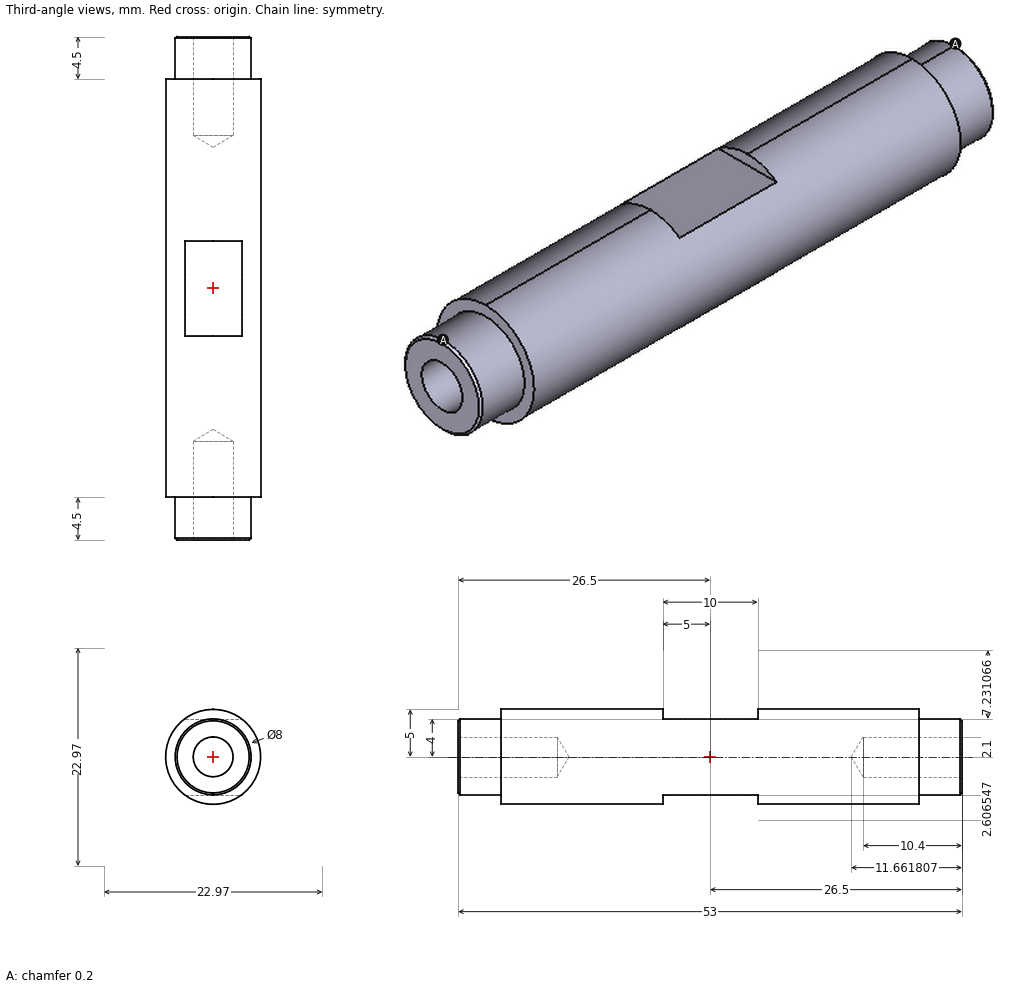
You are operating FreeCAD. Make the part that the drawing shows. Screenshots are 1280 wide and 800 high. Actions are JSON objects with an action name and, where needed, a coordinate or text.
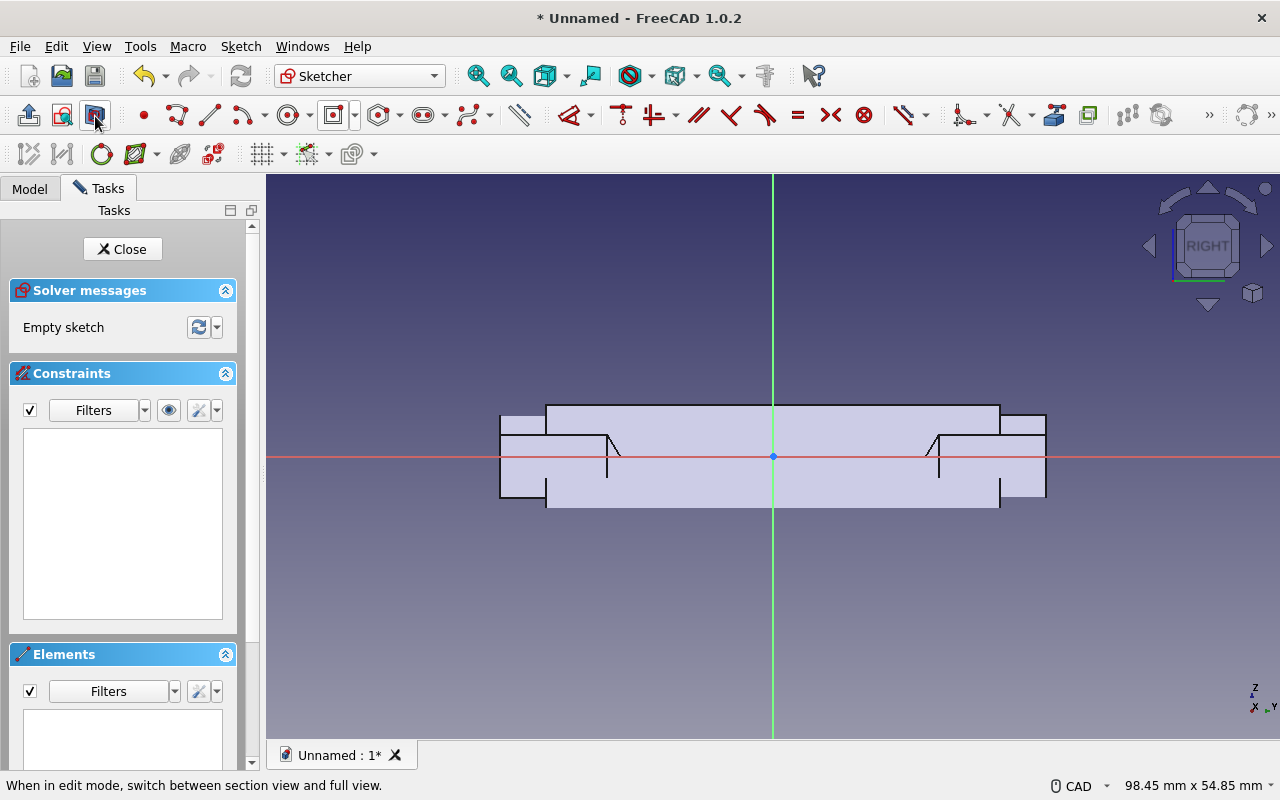
{"action": "scroll", "coordinate": [856, 404], "scroll_direction": "up", "scroll_amount": 3}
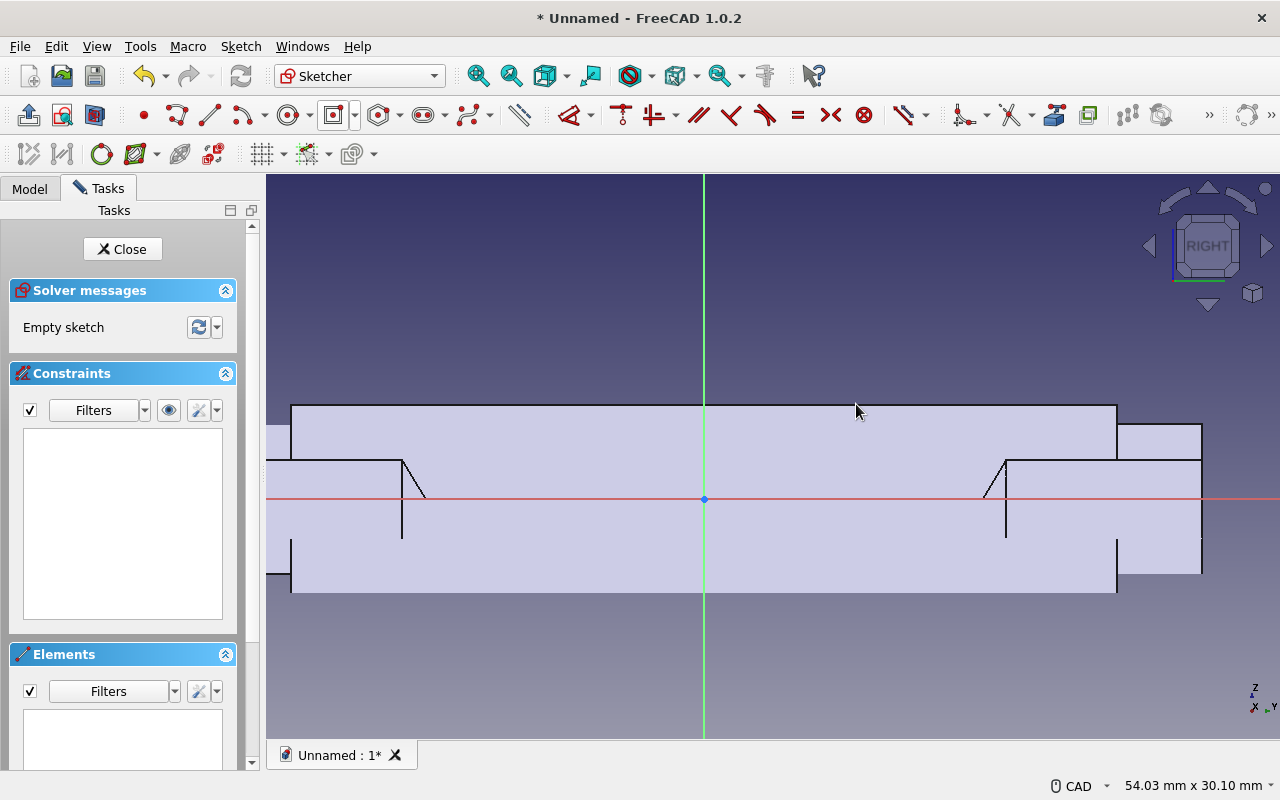
{"action": "left_click", "coordinate": [354, 116]}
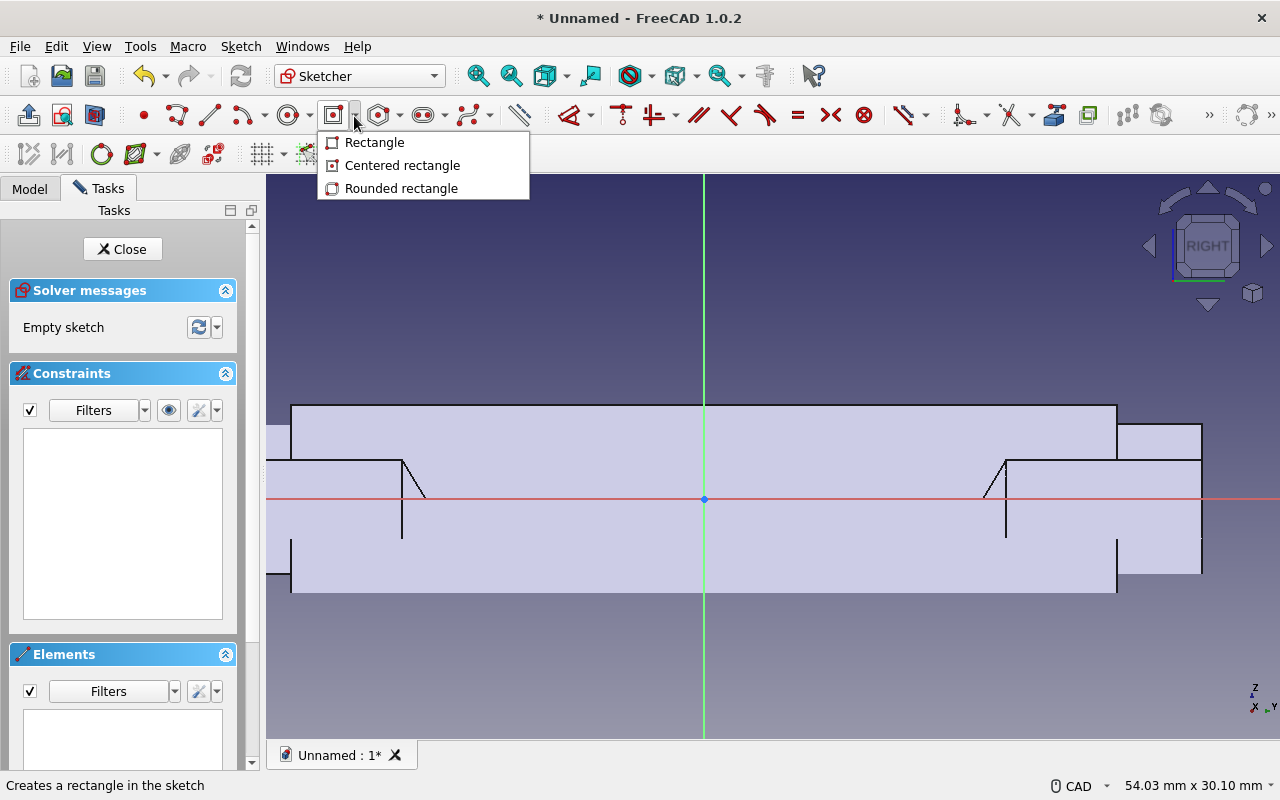
{"action": "left_click", "coordinate": [424, 142]}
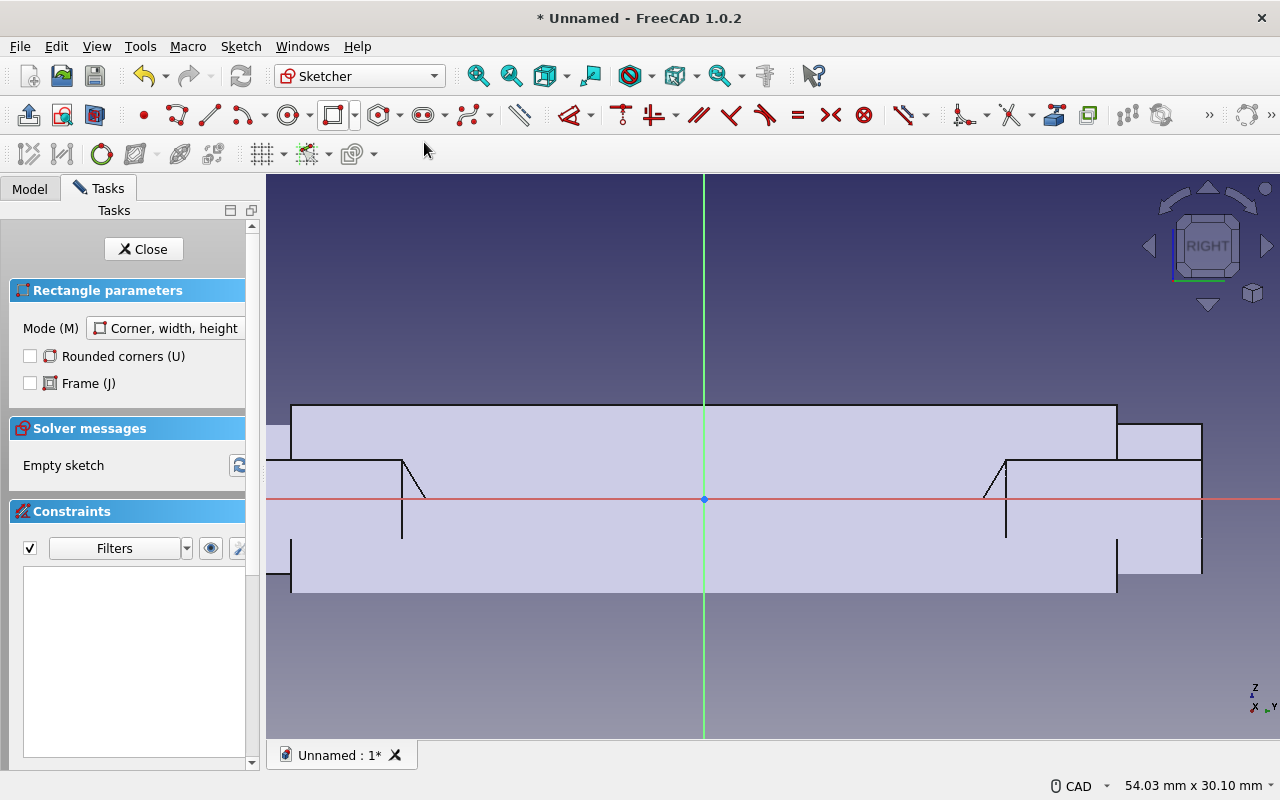
{"action": "left_click", "coordinate": [610, 289]}
{"action": "mouse_move", "coordinate": [798, 424]}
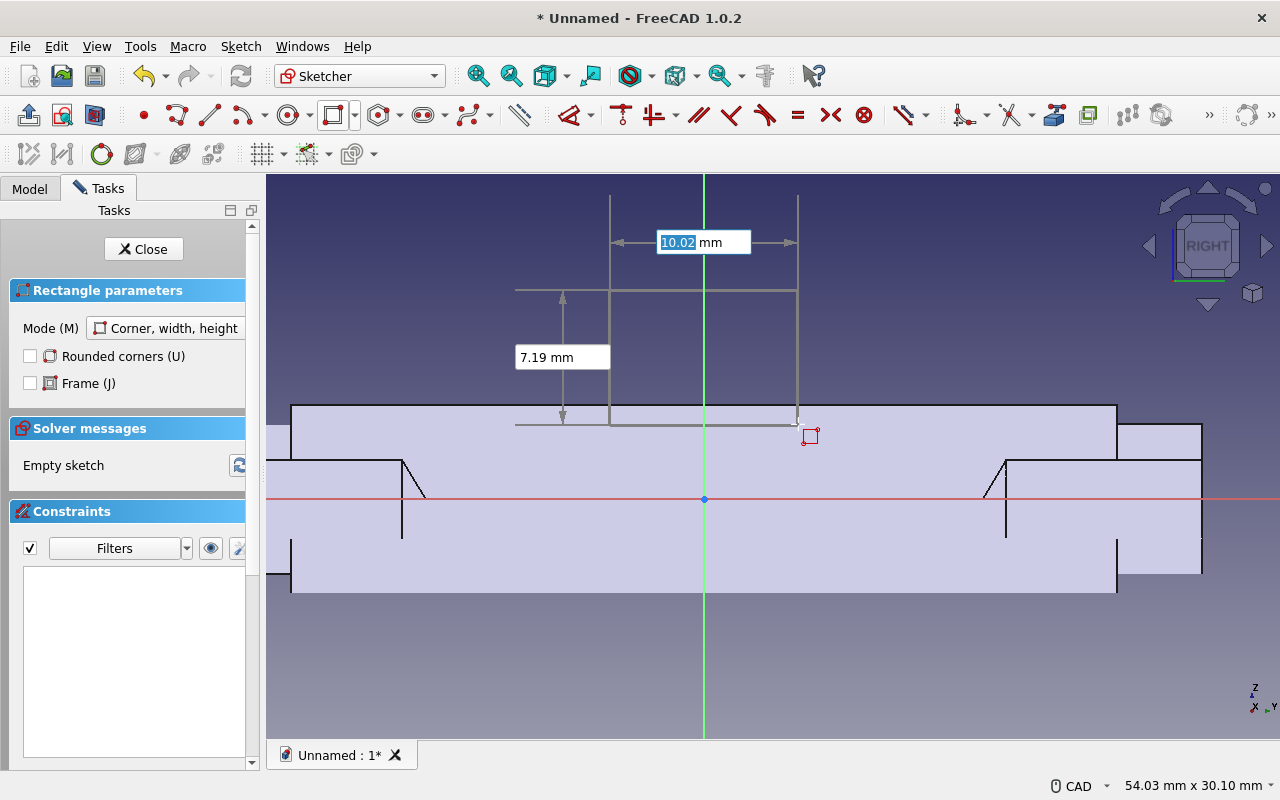
{"action": "type", "text": "10"}
{"action": "key", "text": "Tab"}
{"action": "type", "text": "7.231066"}
{"action": "key", "text": "Return"}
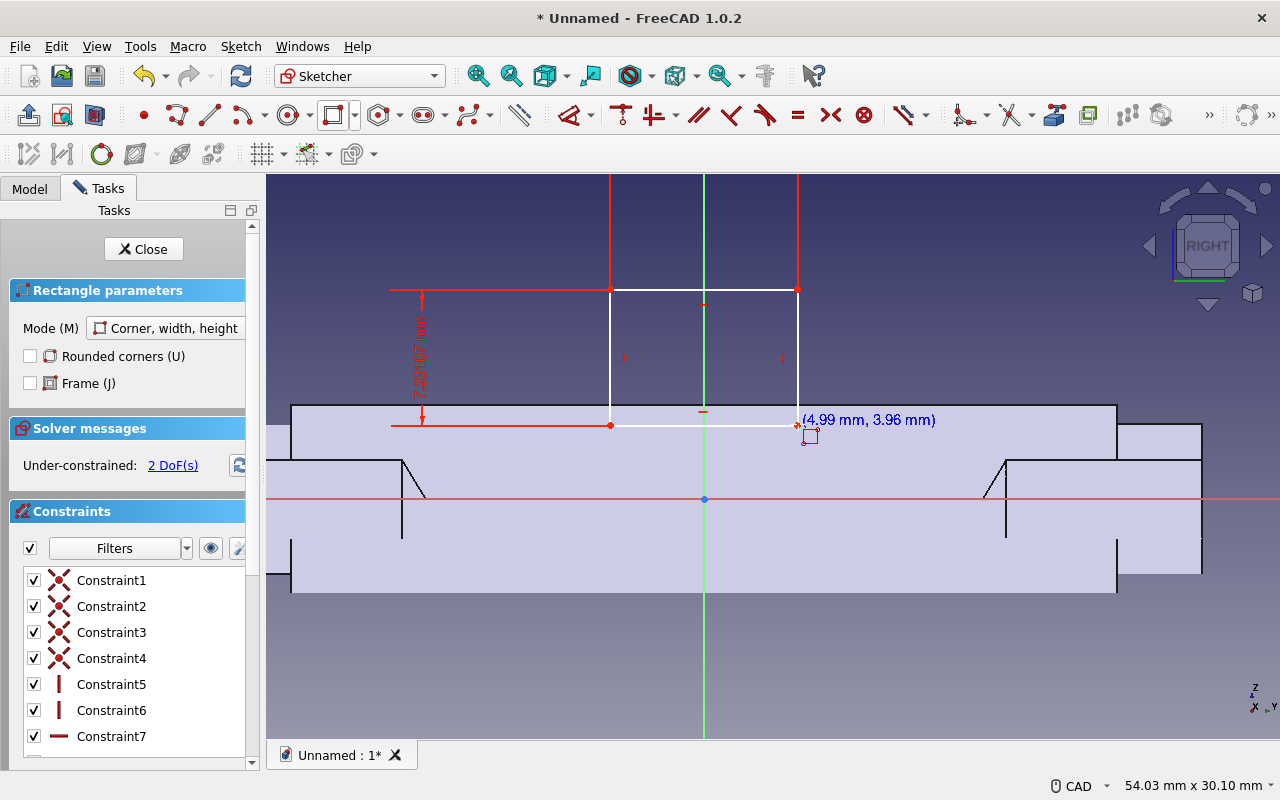
{"action": "left_click", "coordinate": [610, 574]}
{"action": "mouse_move", "coordinate": [798, 623]}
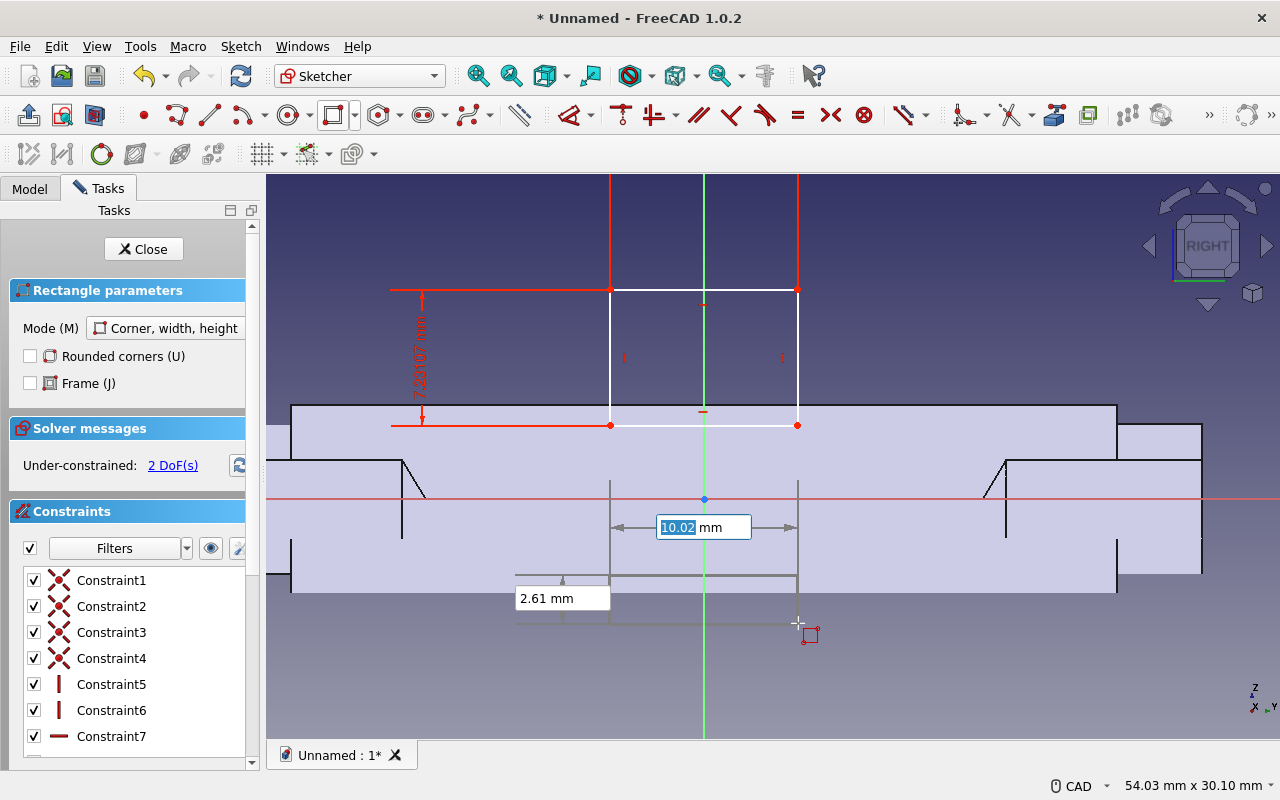
{"action": "type", "text": "10"}
{"action": "key", "text": "Tab"}
{"action": "type", "text": "2.606547"}
{"action": "key", "text": "Return"}
{"action": "key", "text": "Escape"}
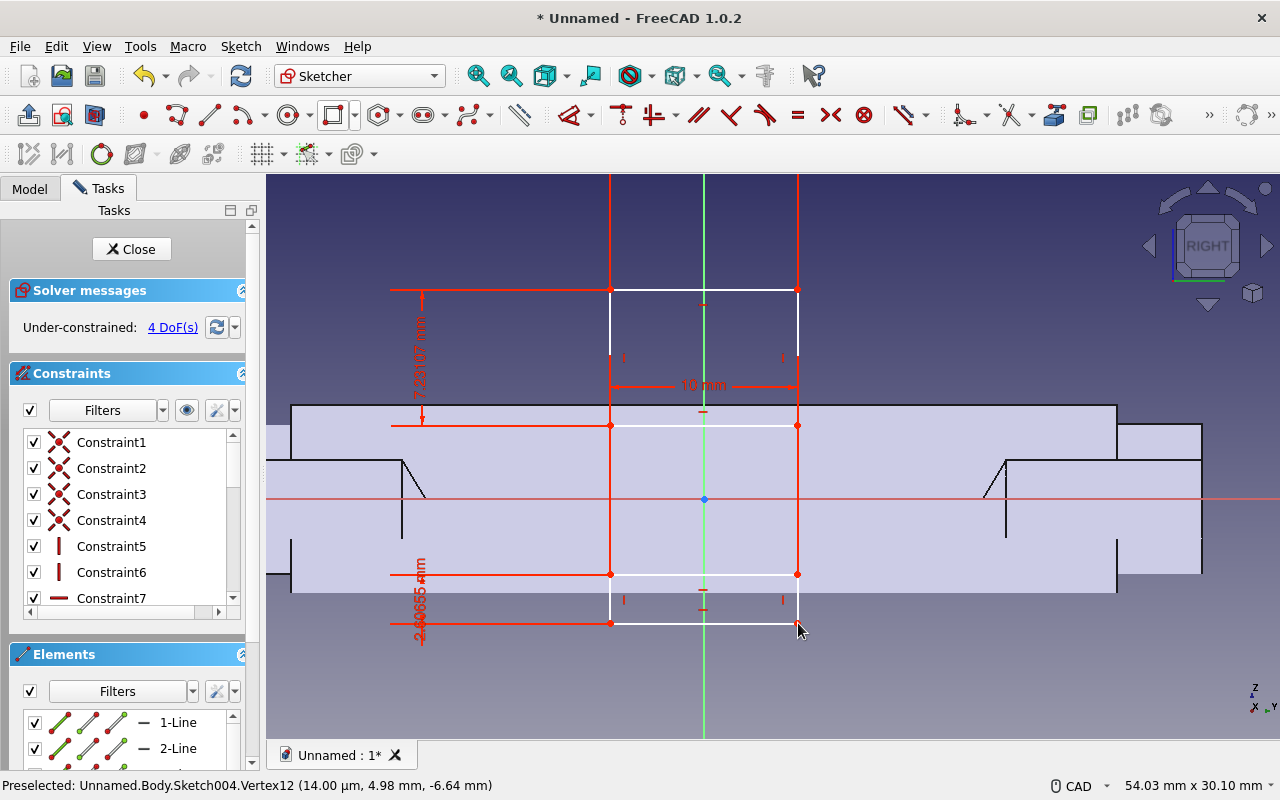
{"action": "left_click", "coordinate": [610, 426]}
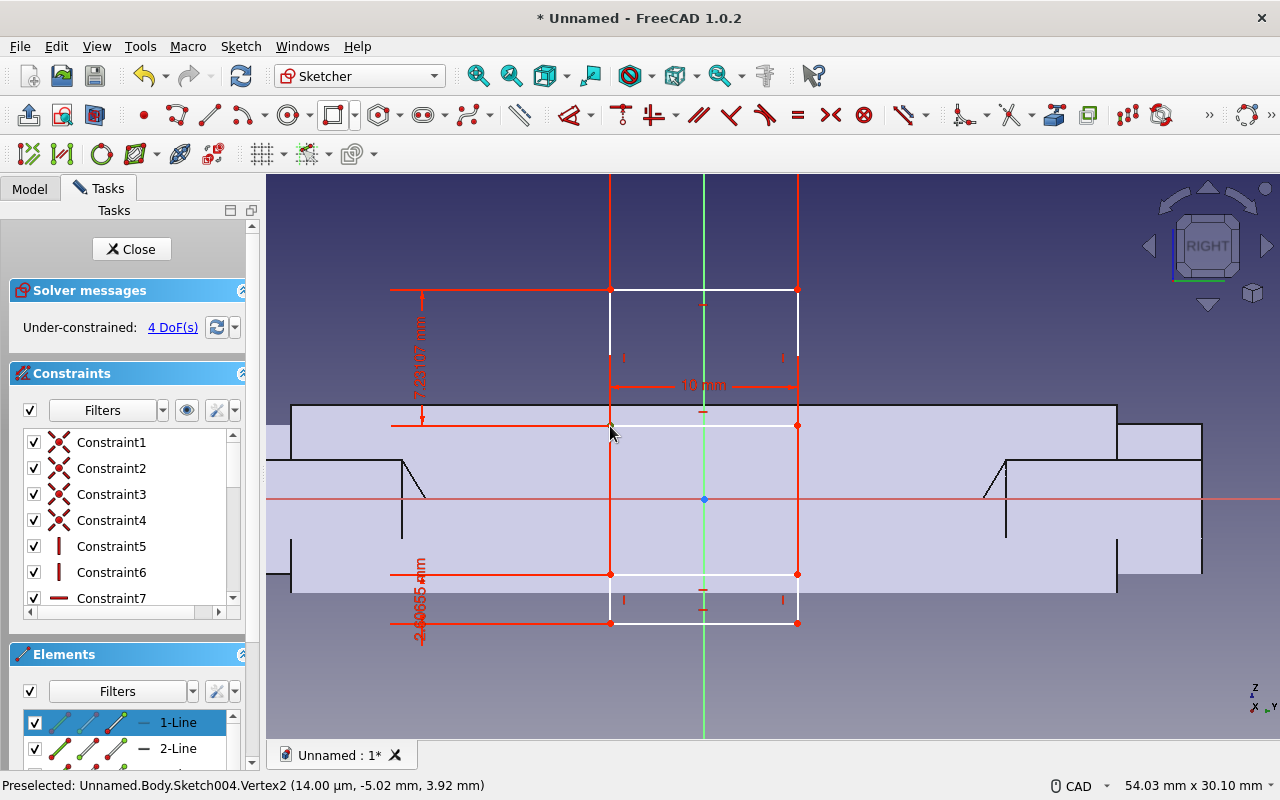
{"action": "left_click", "coordinate": [610, 575]}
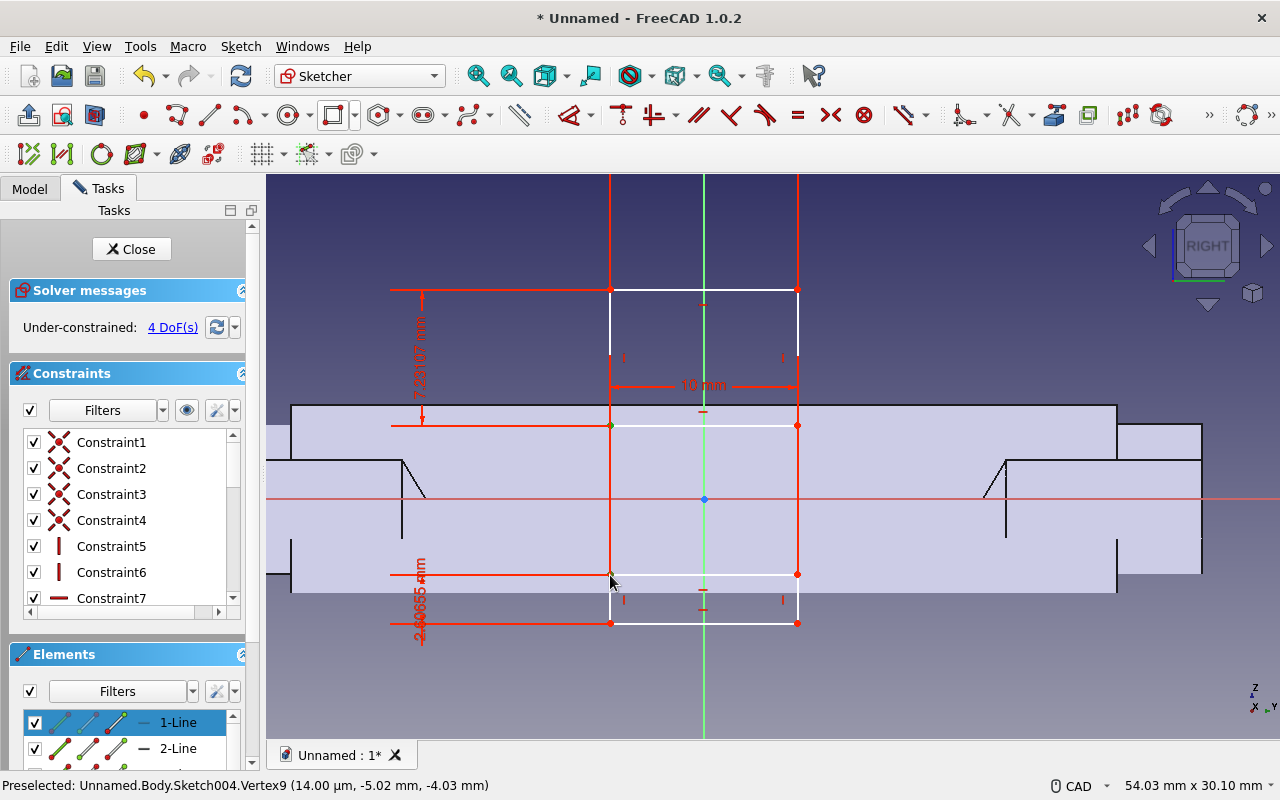
{"action": "left_click", "coordinate": [353, 499]}